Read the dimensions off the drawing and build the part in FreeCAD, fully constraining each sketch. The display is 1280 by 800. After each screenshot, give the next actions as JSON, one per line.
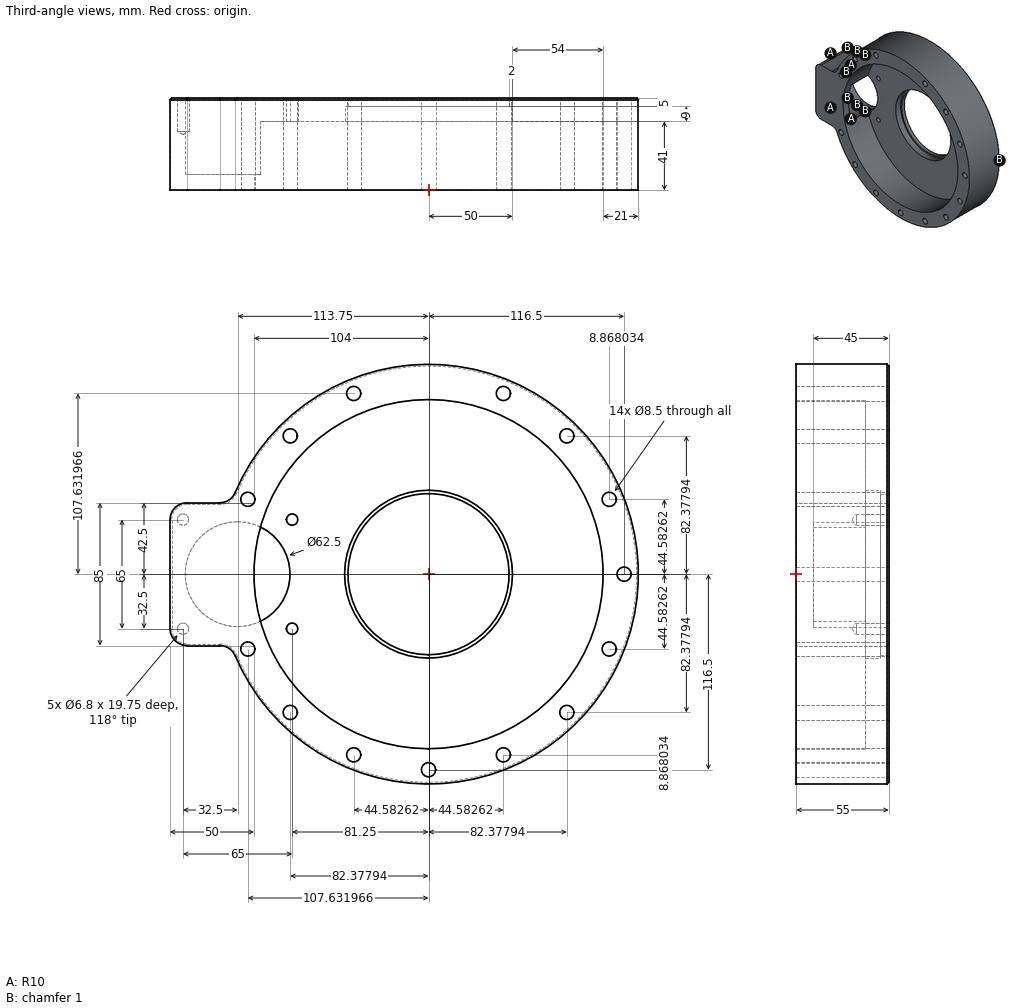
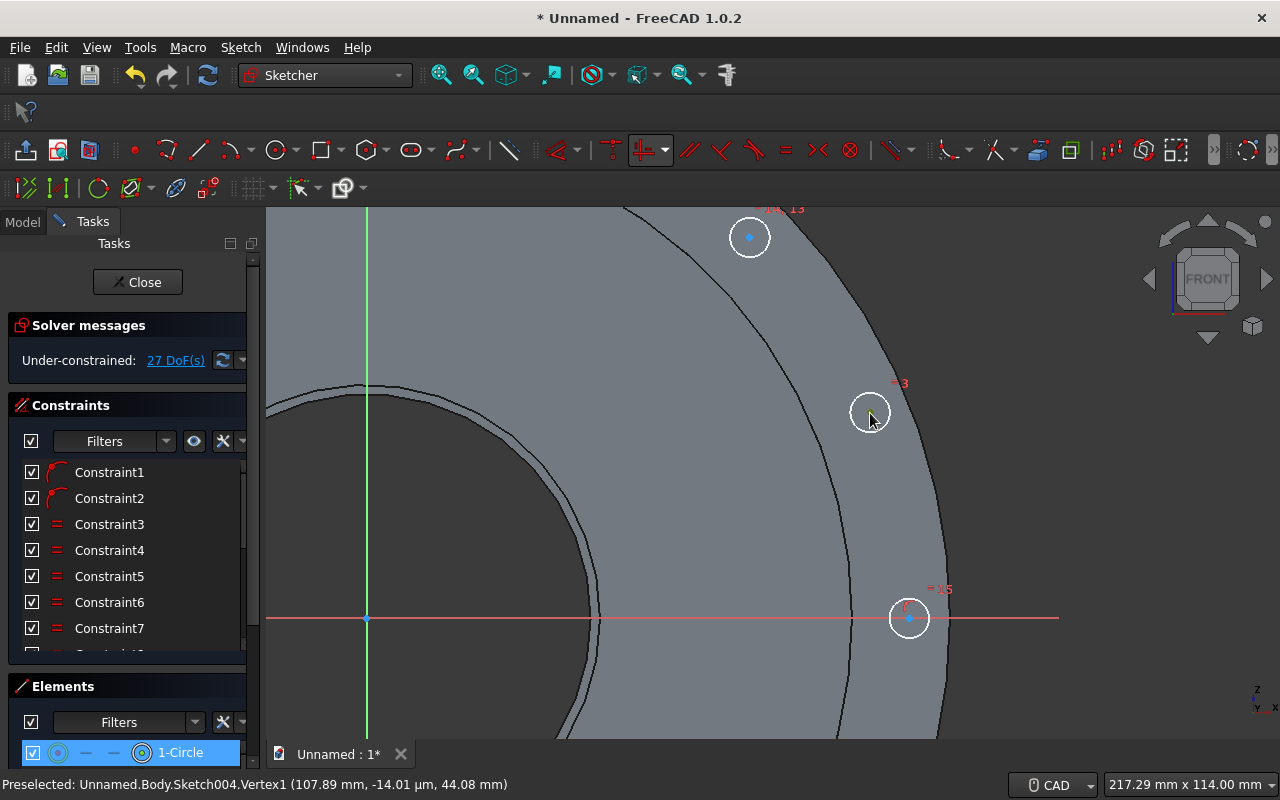
{"action": "scroll", "coordinate": [841, 401], "scroll_direction": "down", "scroll_amount": 6}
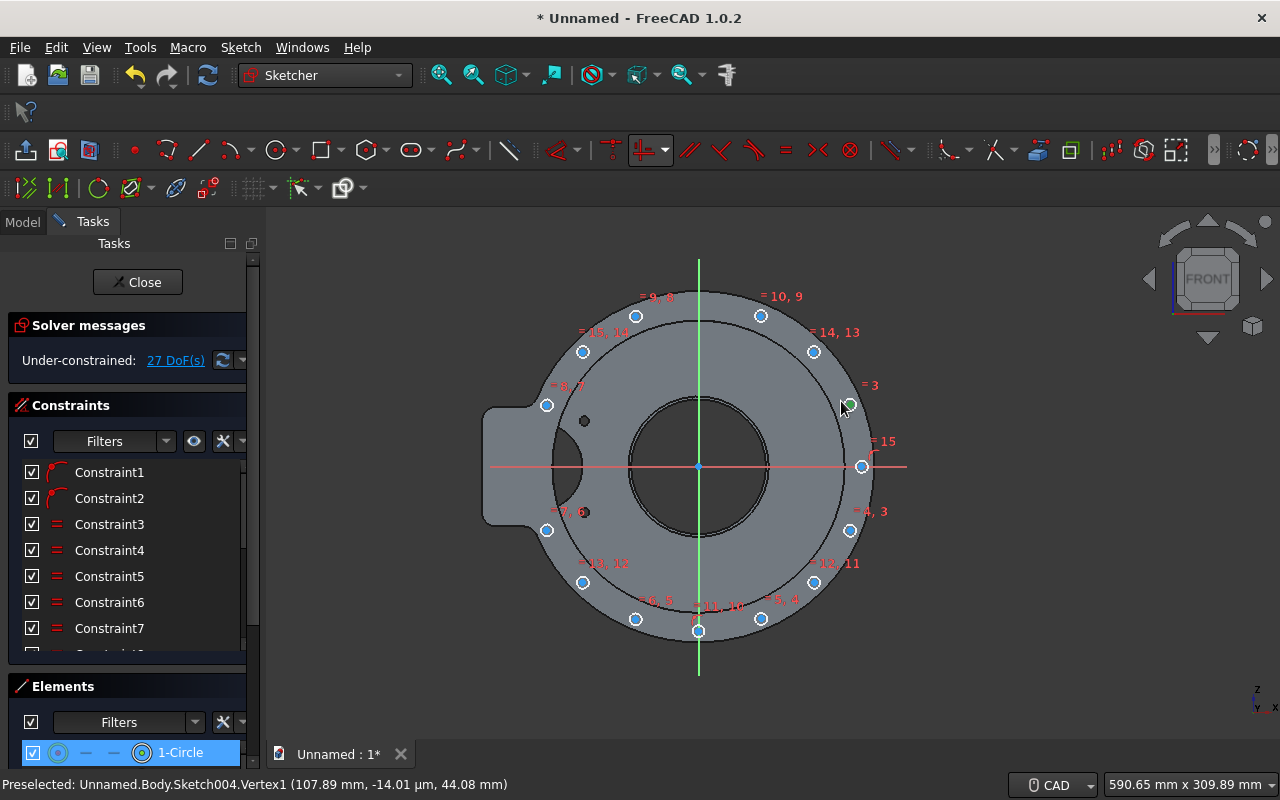
{"action": "left_click", "coordinate": [850, 531]}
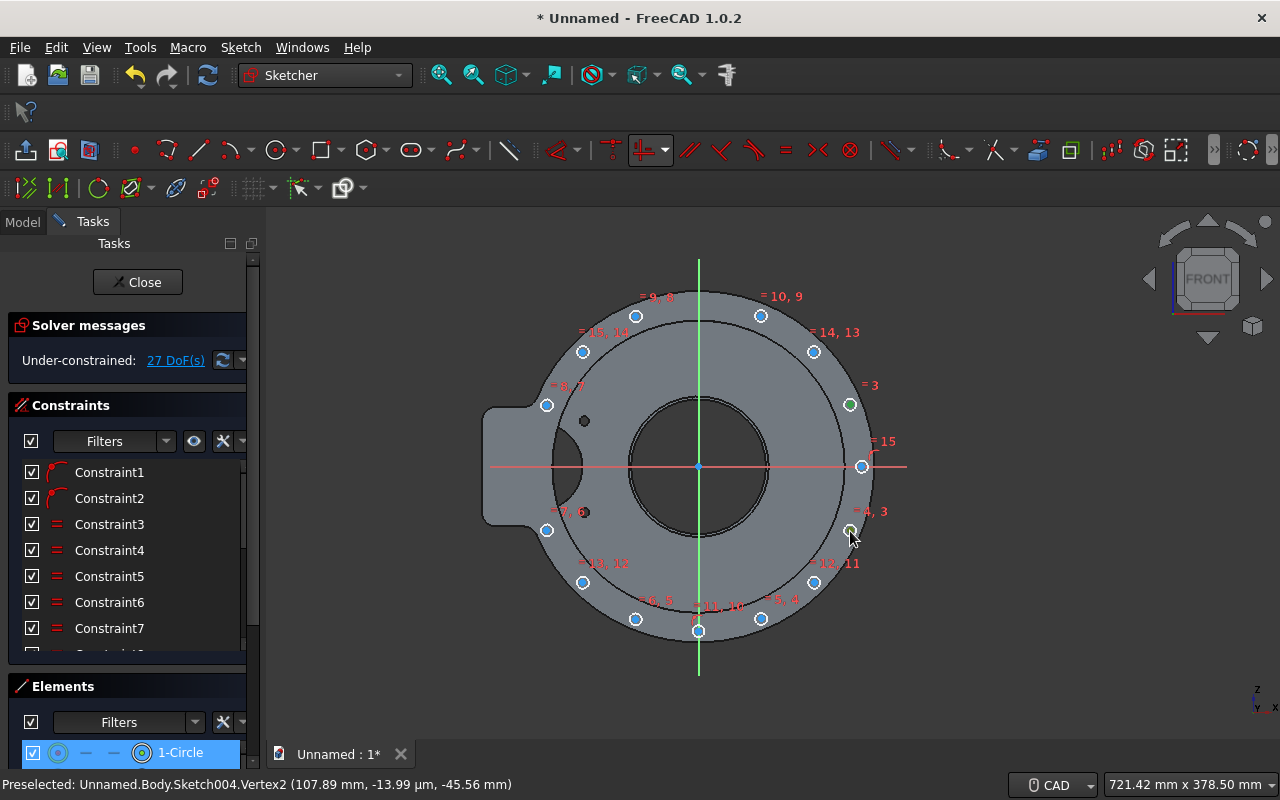
{"action": "key", "text": "v"}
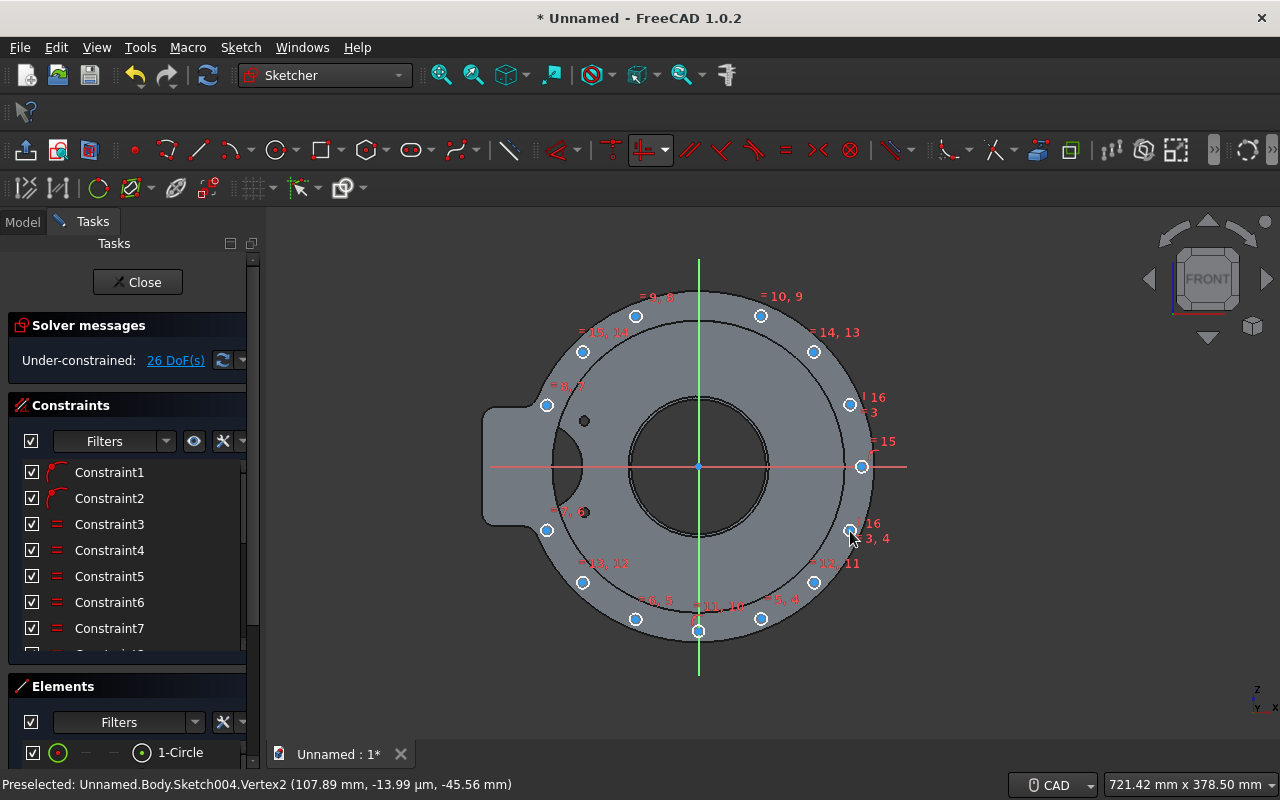
{"action": "left_click", "coordinate": [761, 619]}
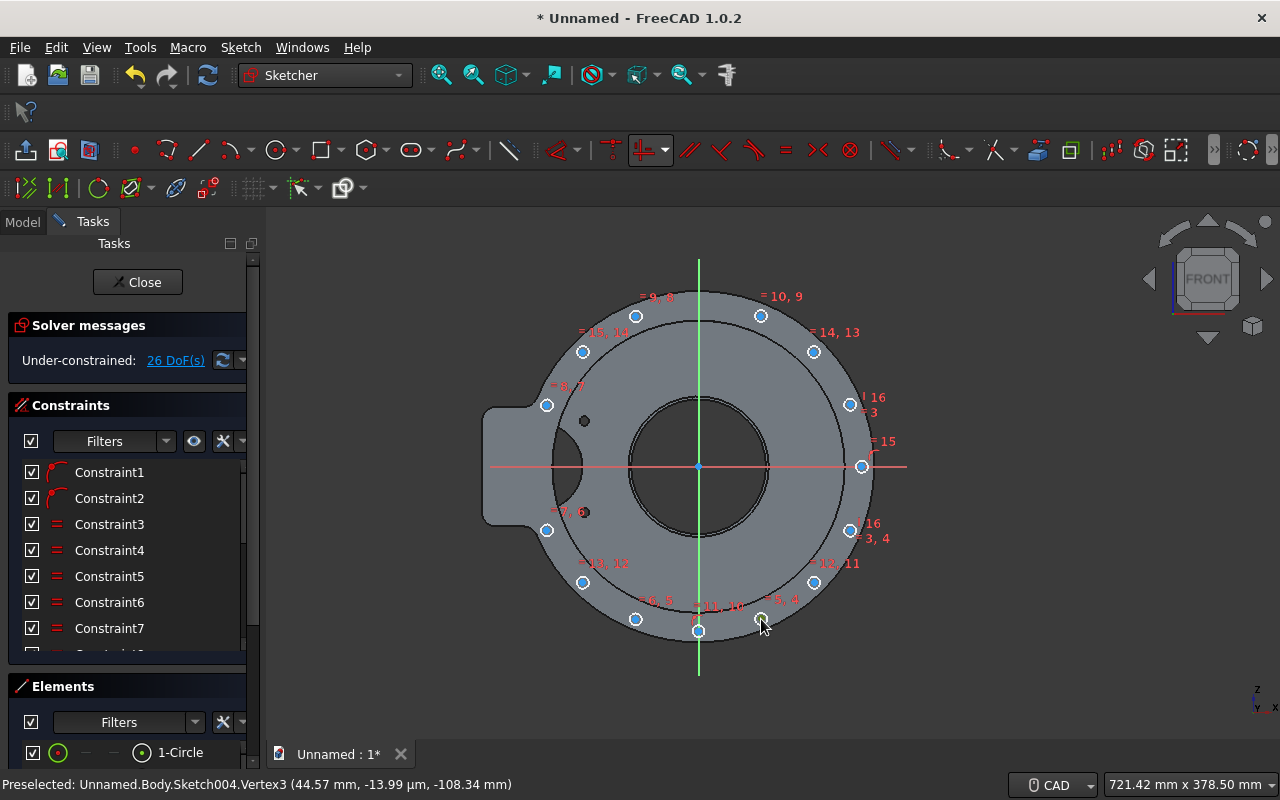
{"action": "left_click", "coordinate": [636, 619]}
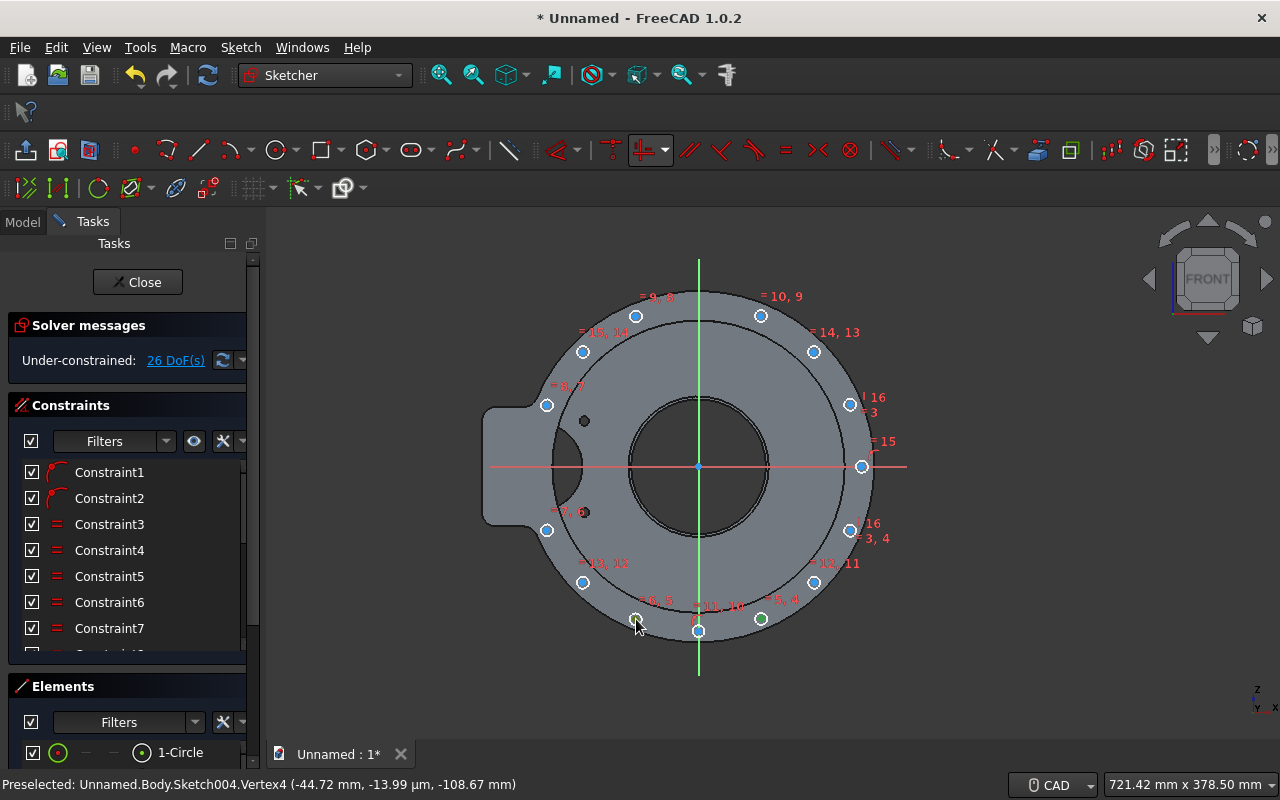
{"action": "left_click", "coordinate": [668, 150]}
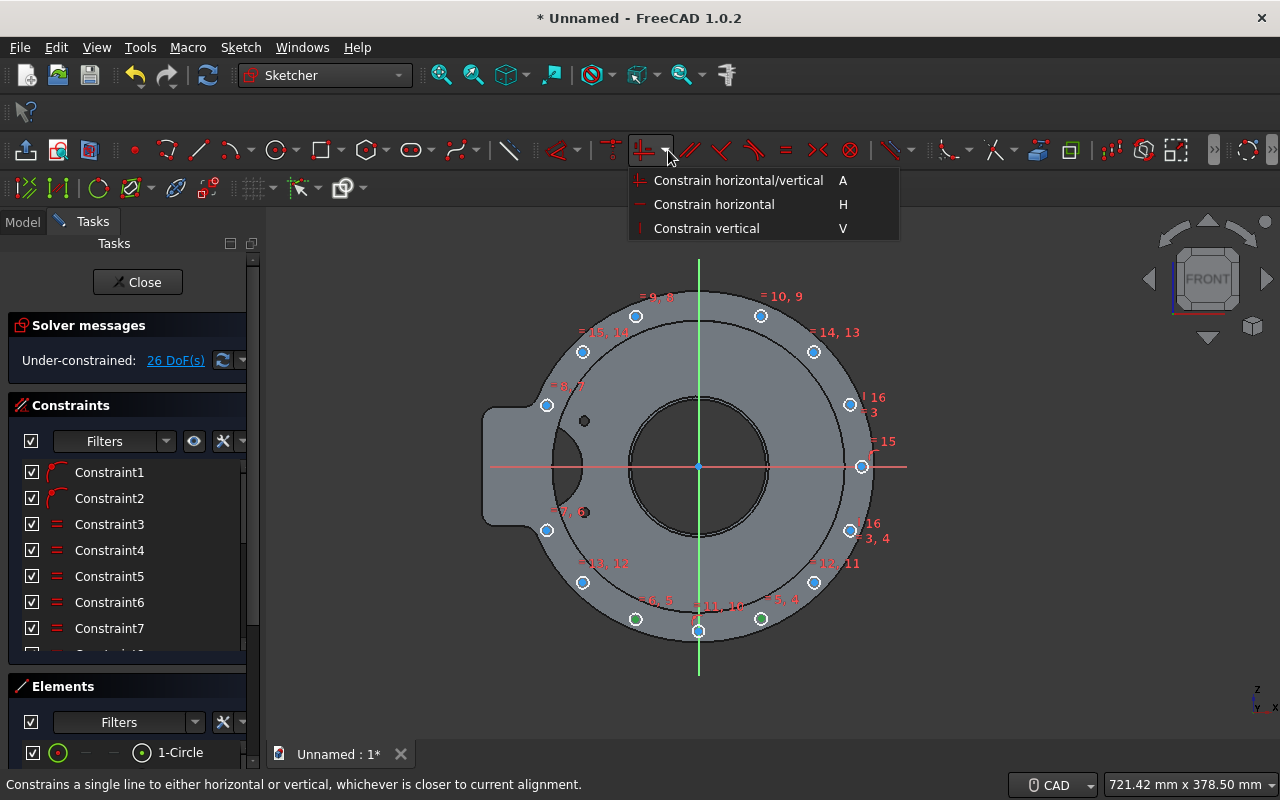
{"action": "left_click", "coordinate": [764, 204]}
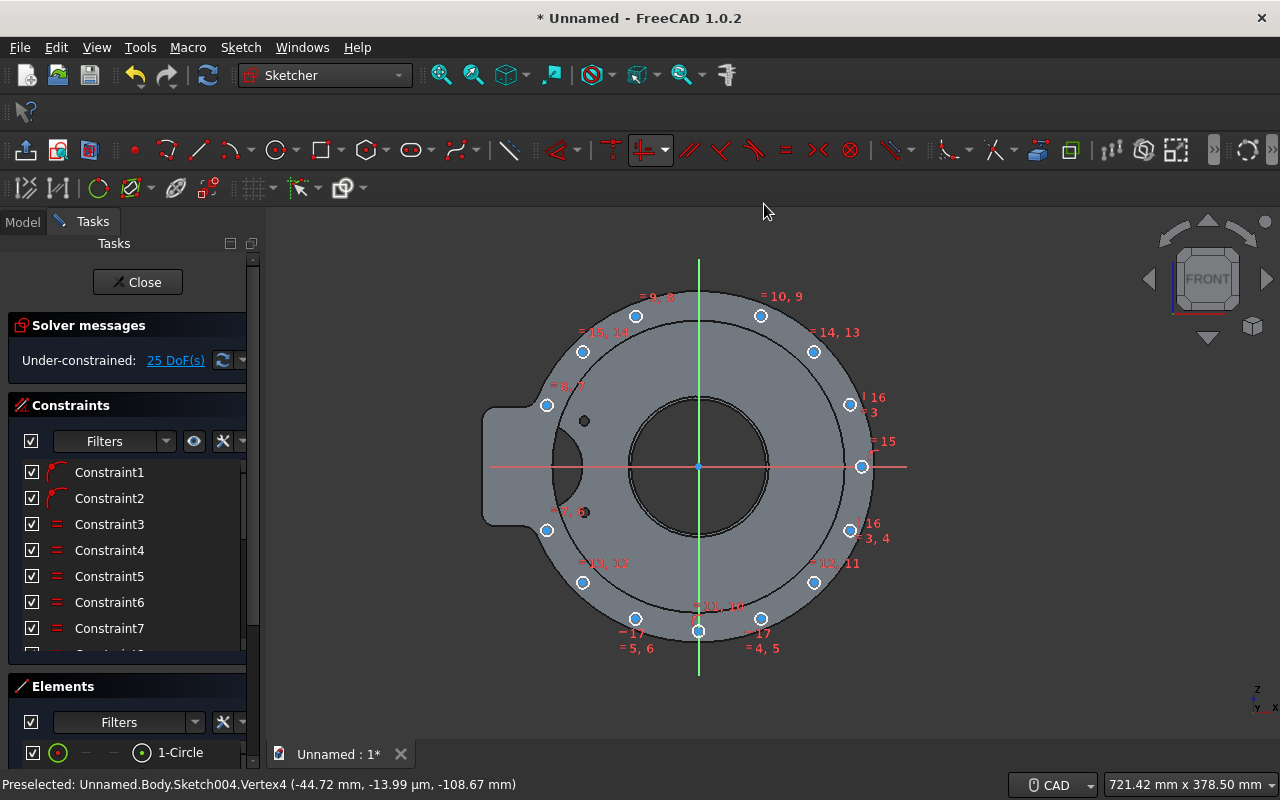
{"action": "left_click", "coordinate": [850, 531]}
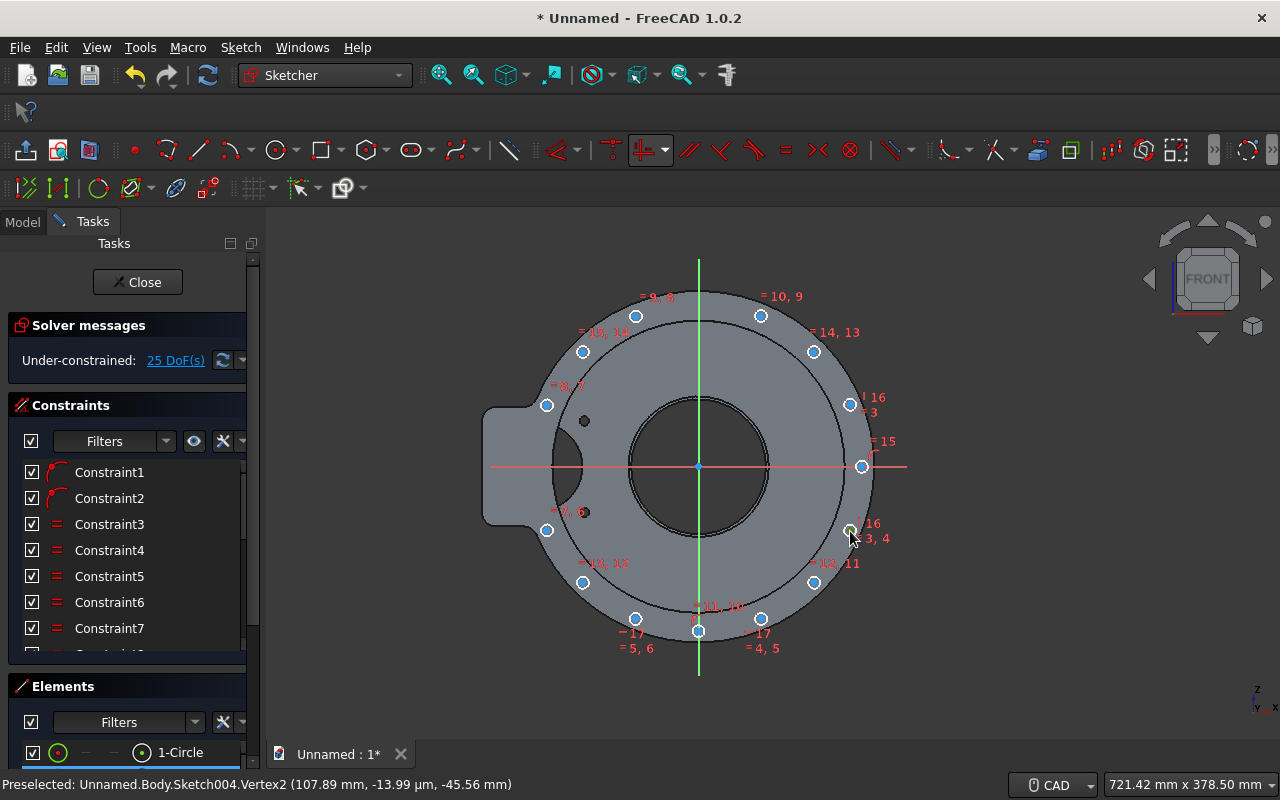
{"action": "left_click", "coordinate": [547, 530]}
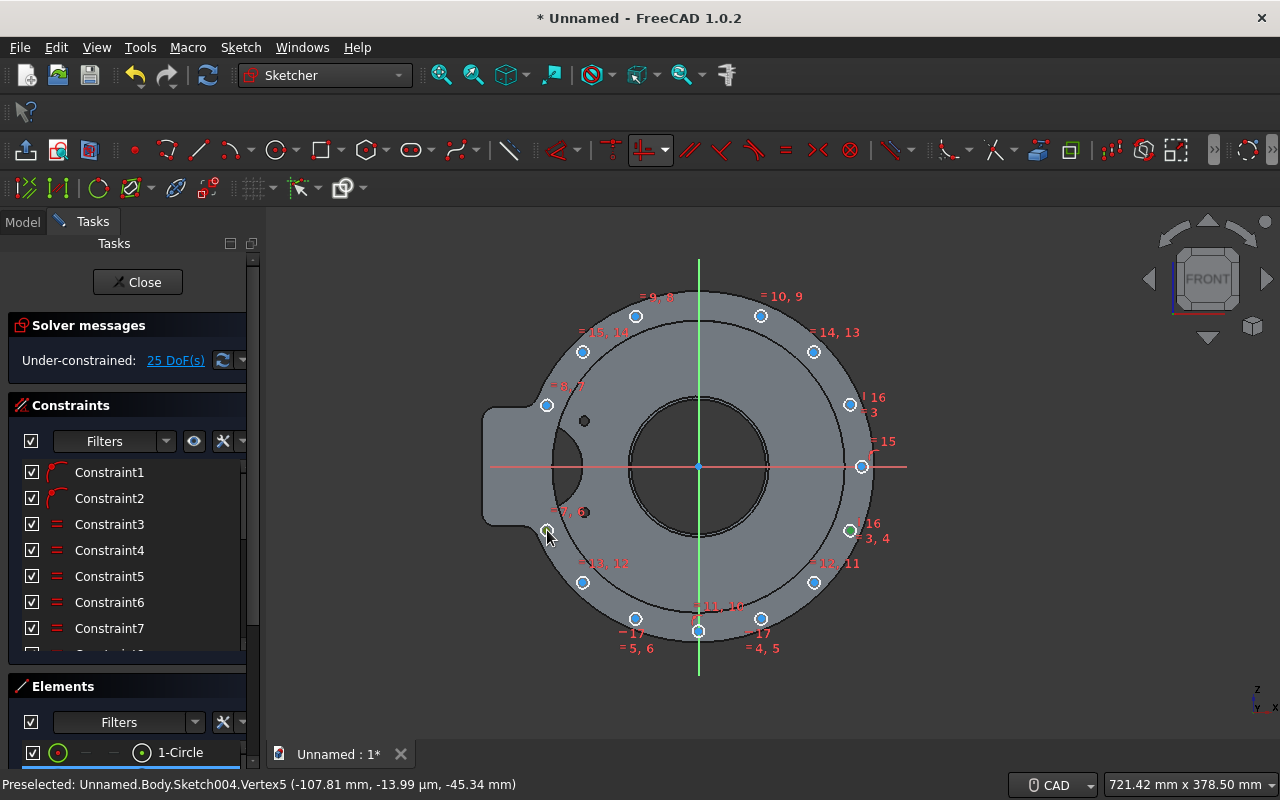
{"action": "key", "text": "h"}